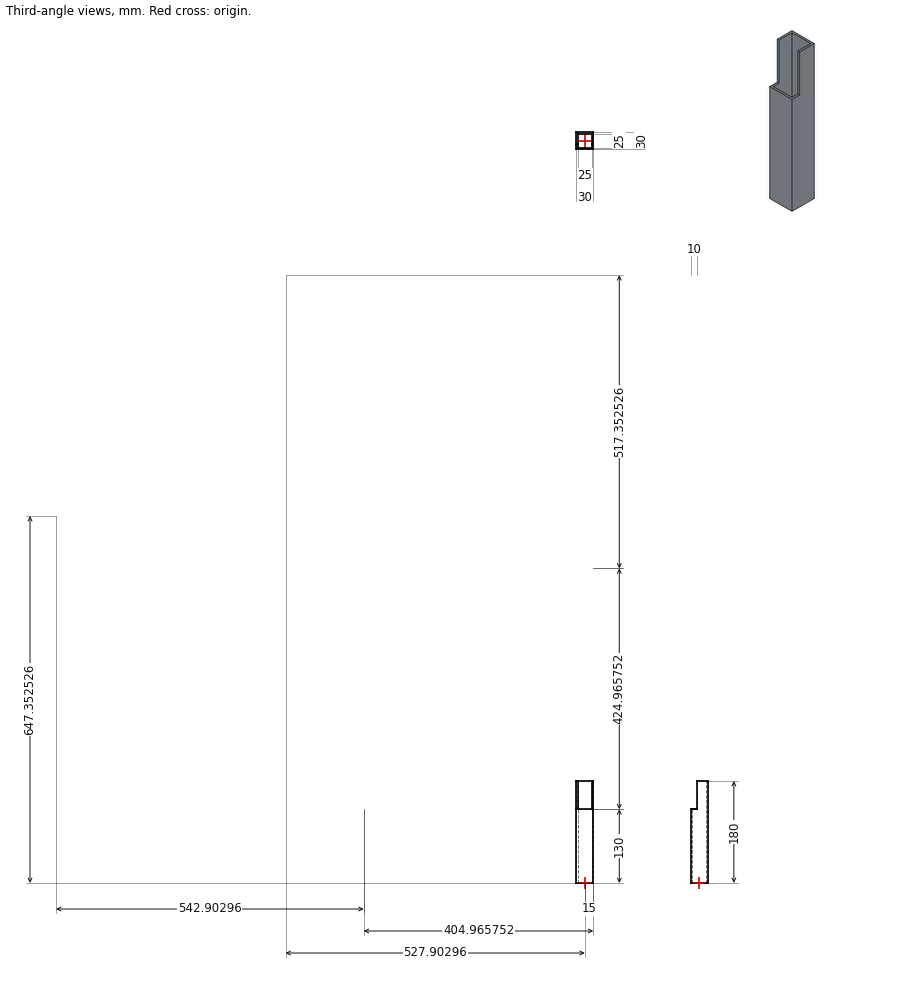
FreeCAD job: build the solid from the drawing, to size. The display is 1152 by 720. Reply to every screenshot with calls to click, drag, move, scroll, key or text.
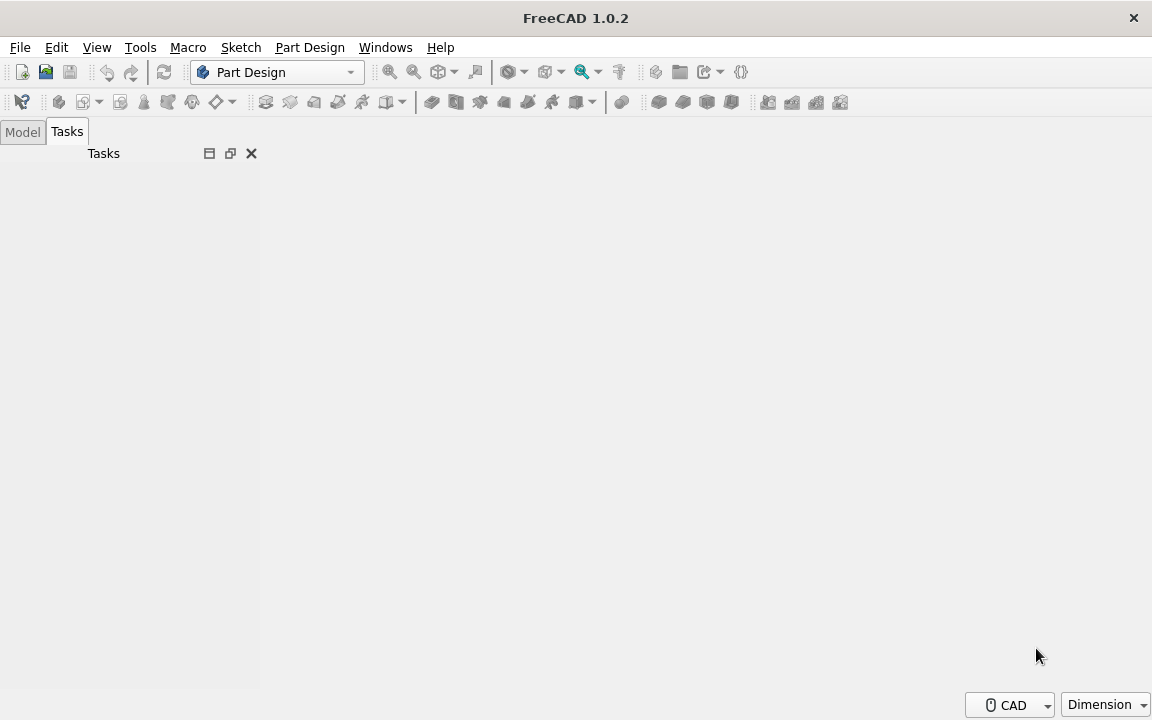
click(22, 72)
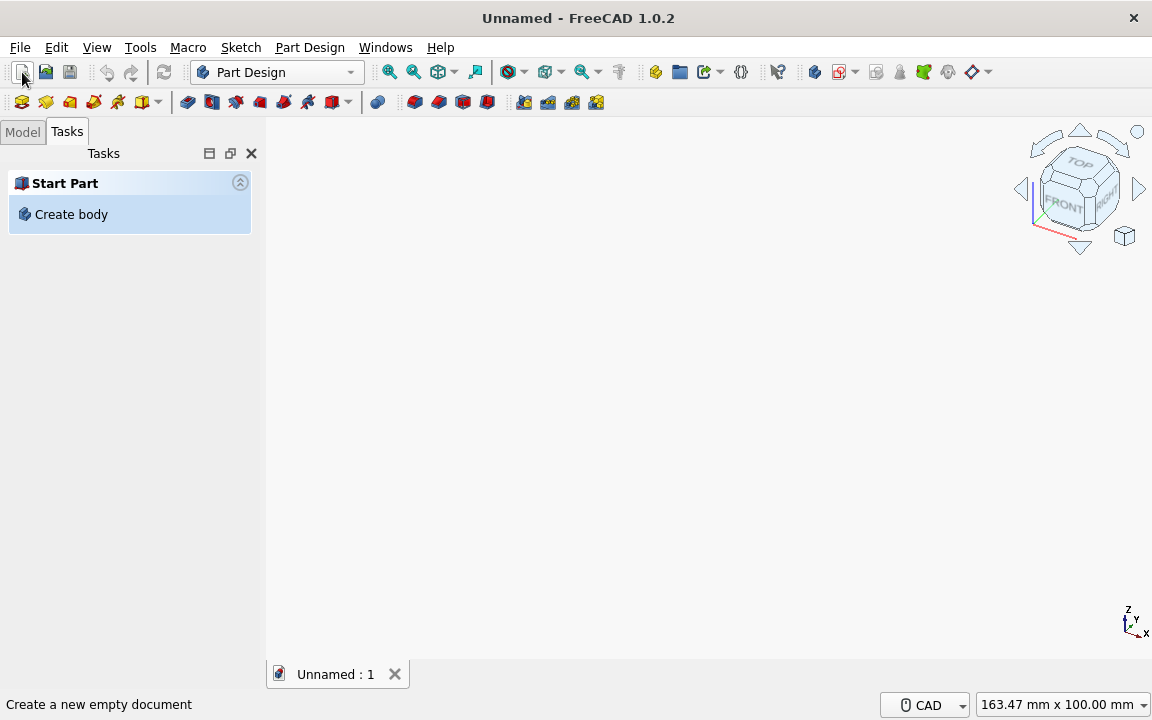
click(840, 72)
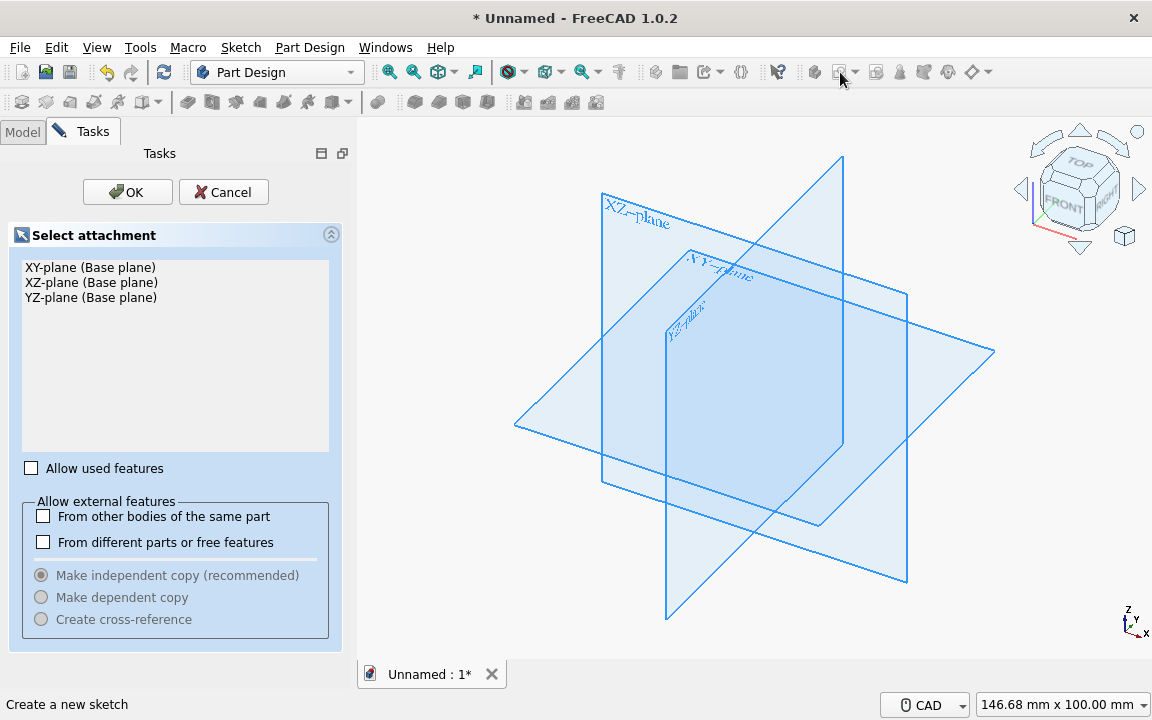
click(82, 268)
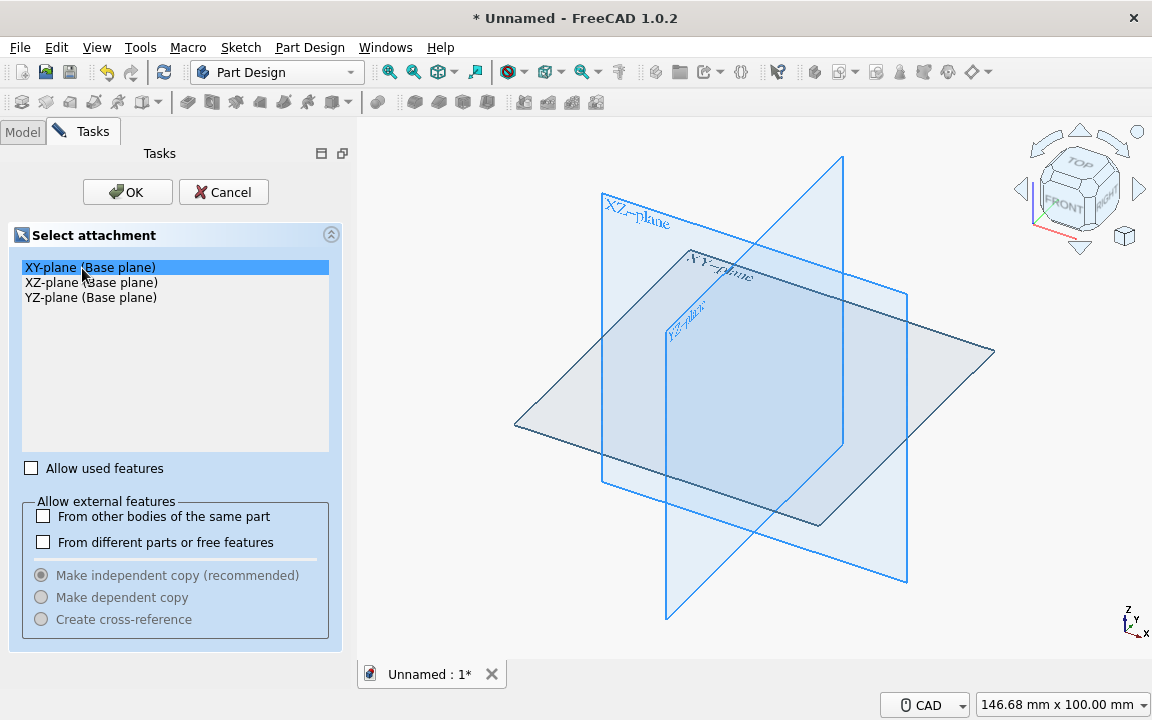
click(128, 192)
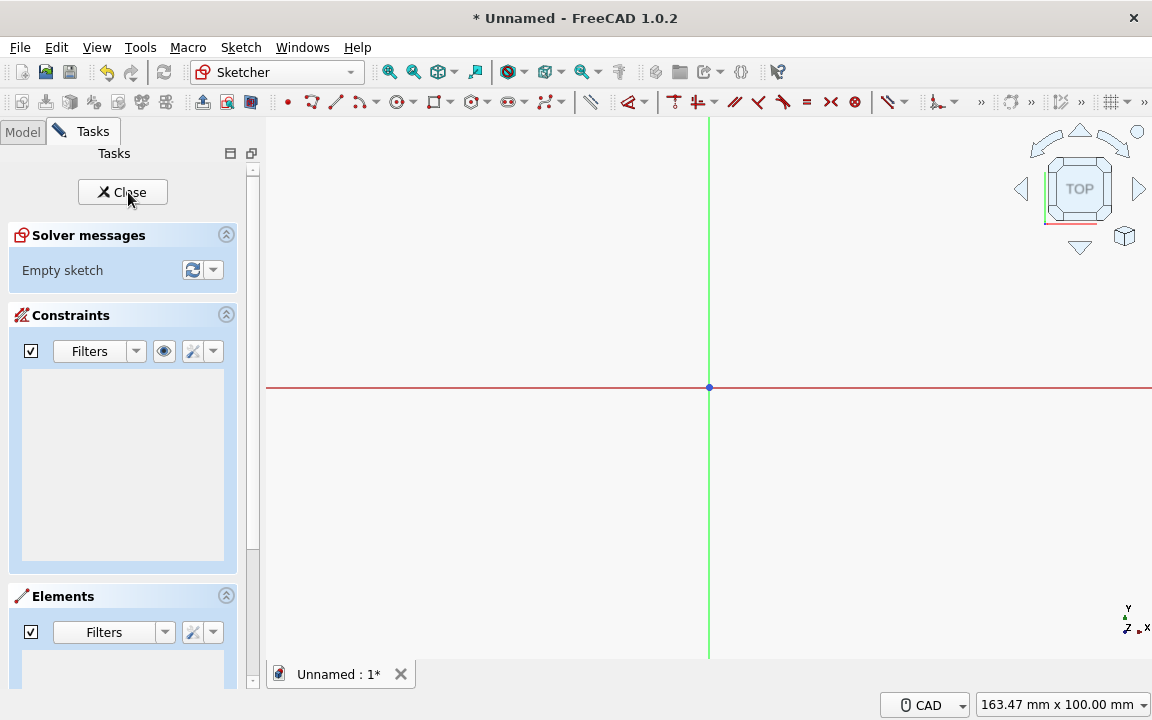
scroll(765, 388, up, 4)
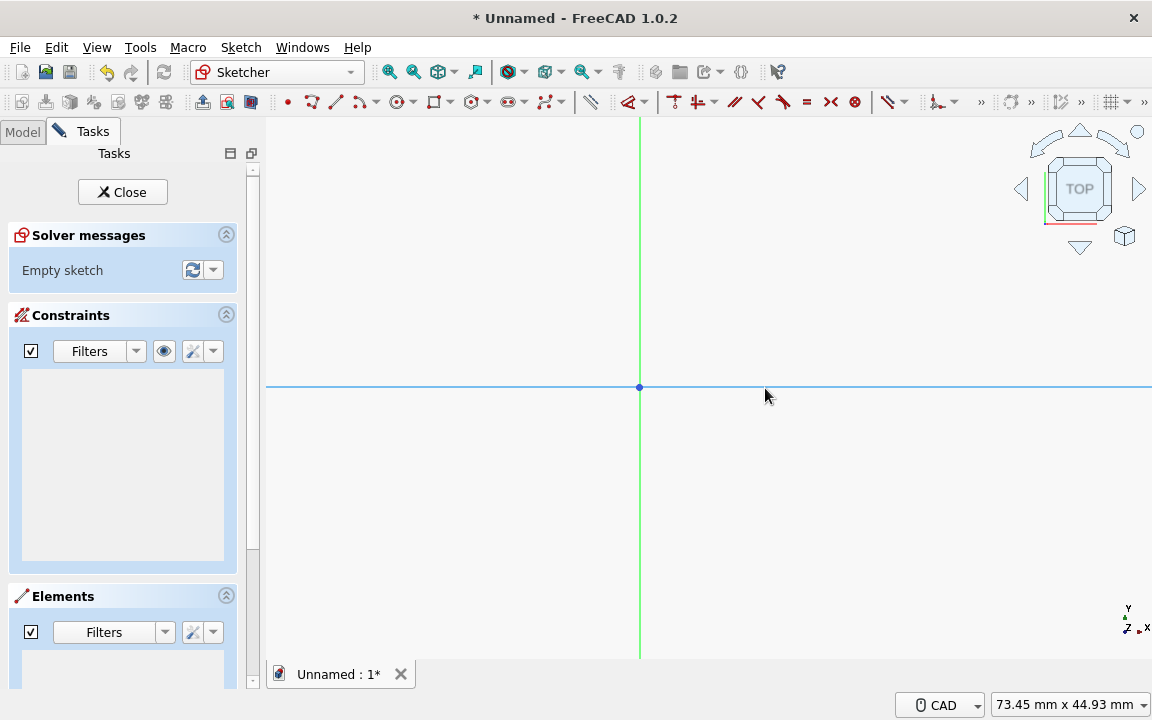
key(g)
key(v)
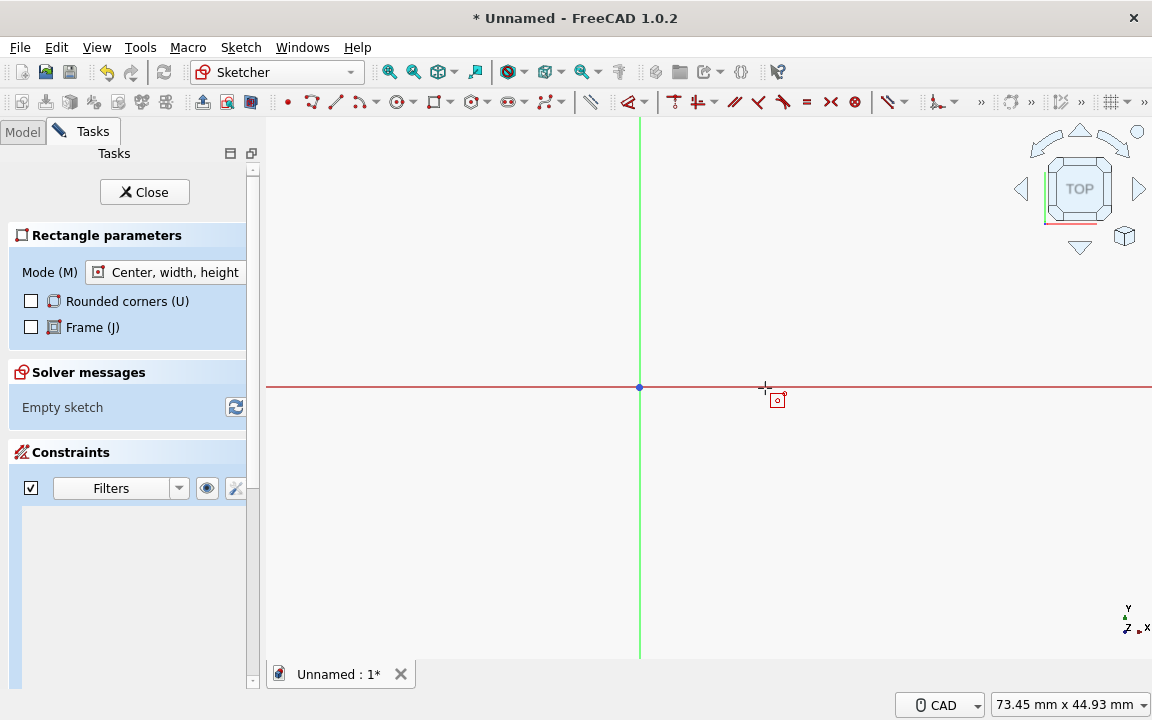
click(640, 387)
move(821, 206)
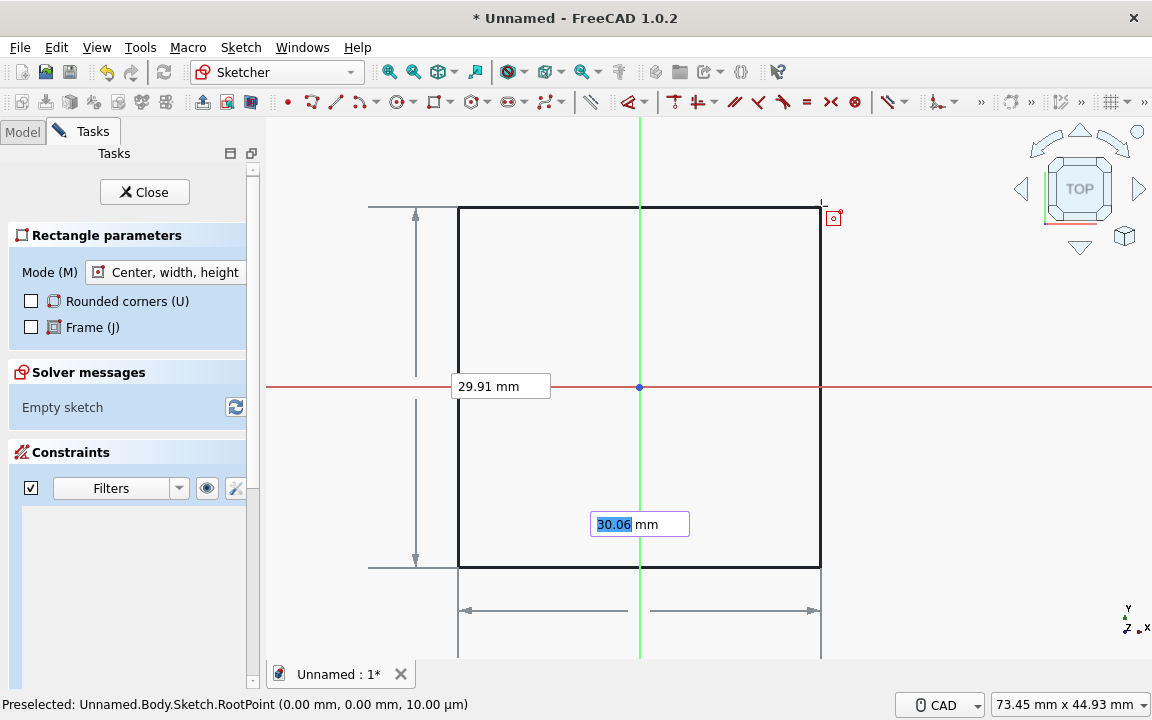
text(30)
key(Tab)
text(30)
key(Return)
key(Escape)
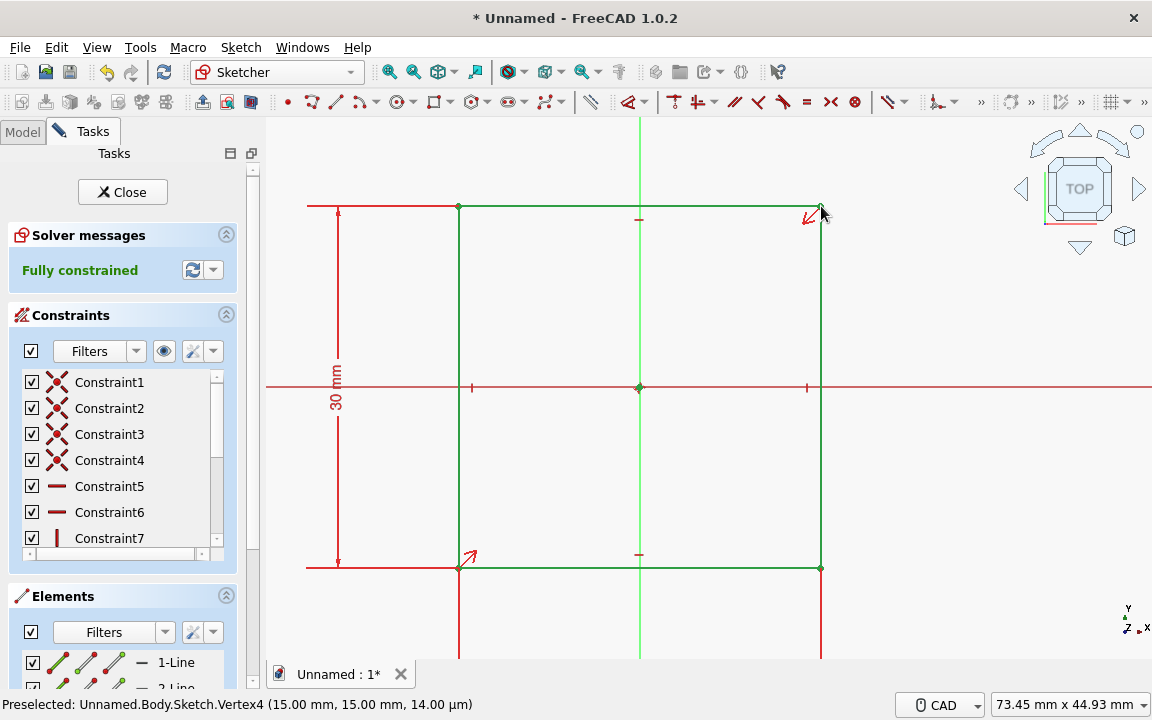
click(123, 192)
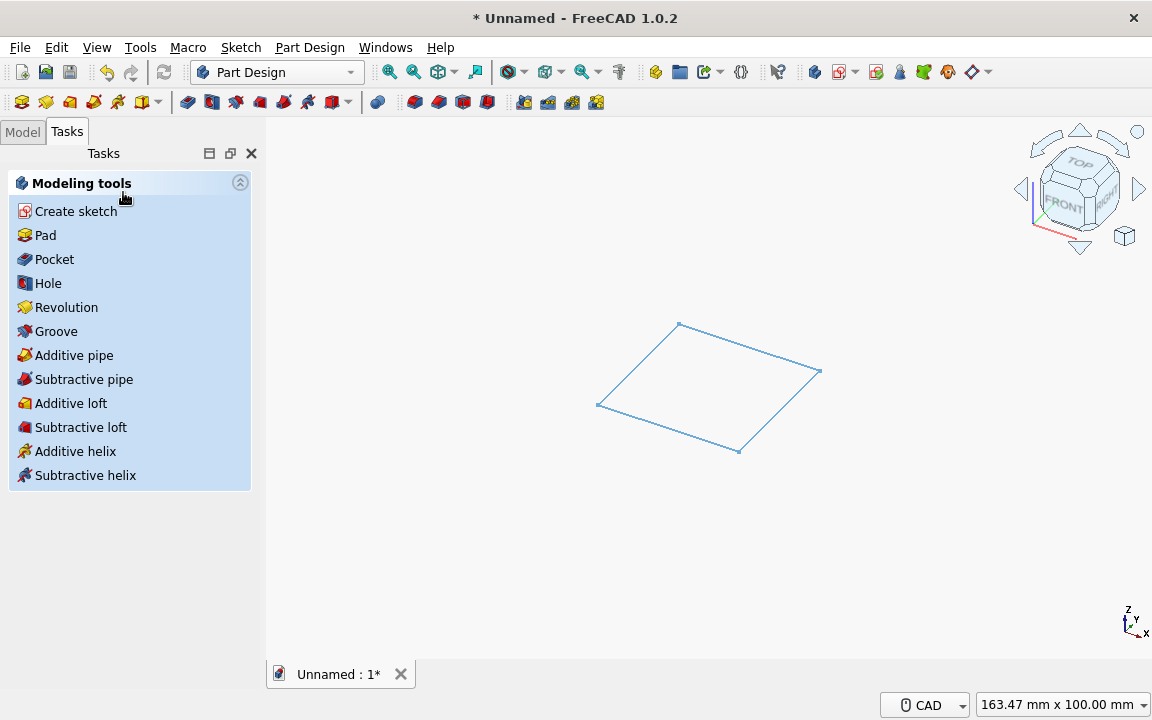
click(22, 102)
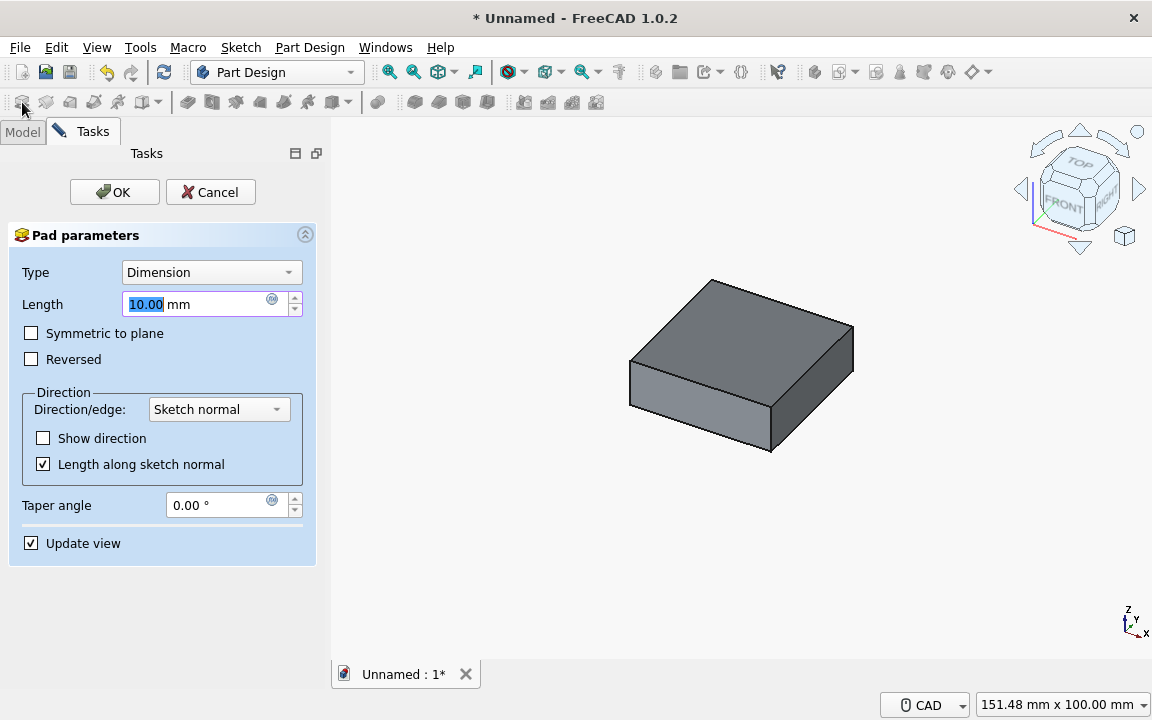
text(180)
key(Tab)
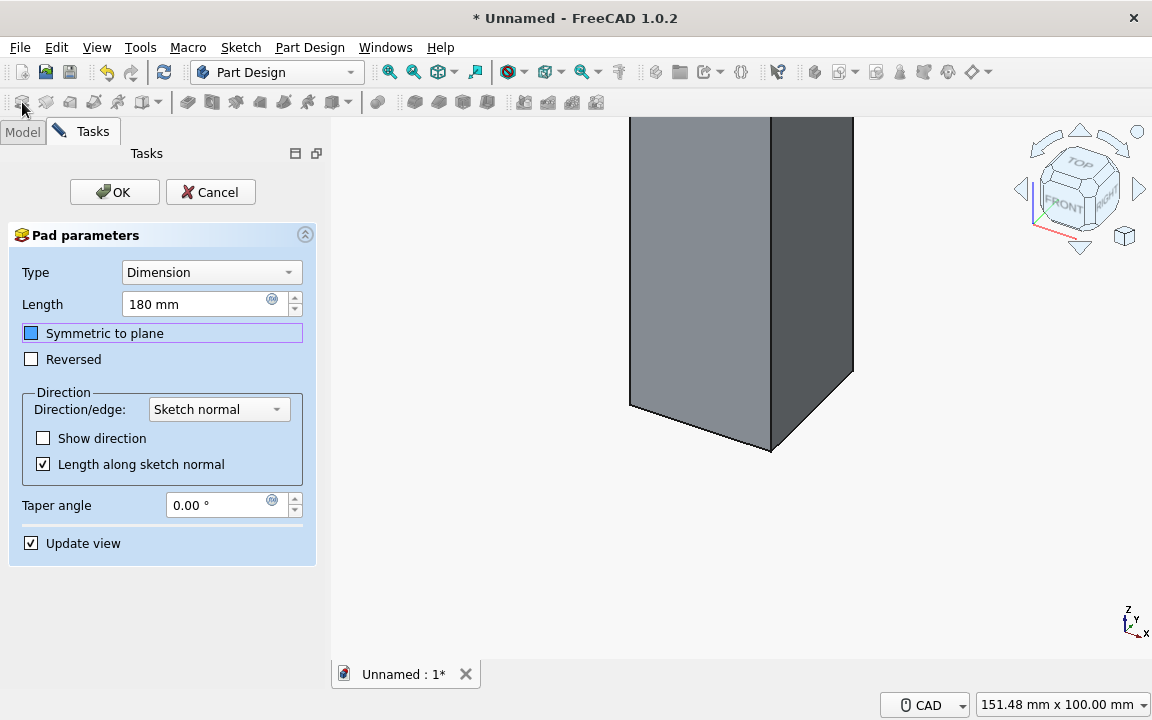
click(115, 192)